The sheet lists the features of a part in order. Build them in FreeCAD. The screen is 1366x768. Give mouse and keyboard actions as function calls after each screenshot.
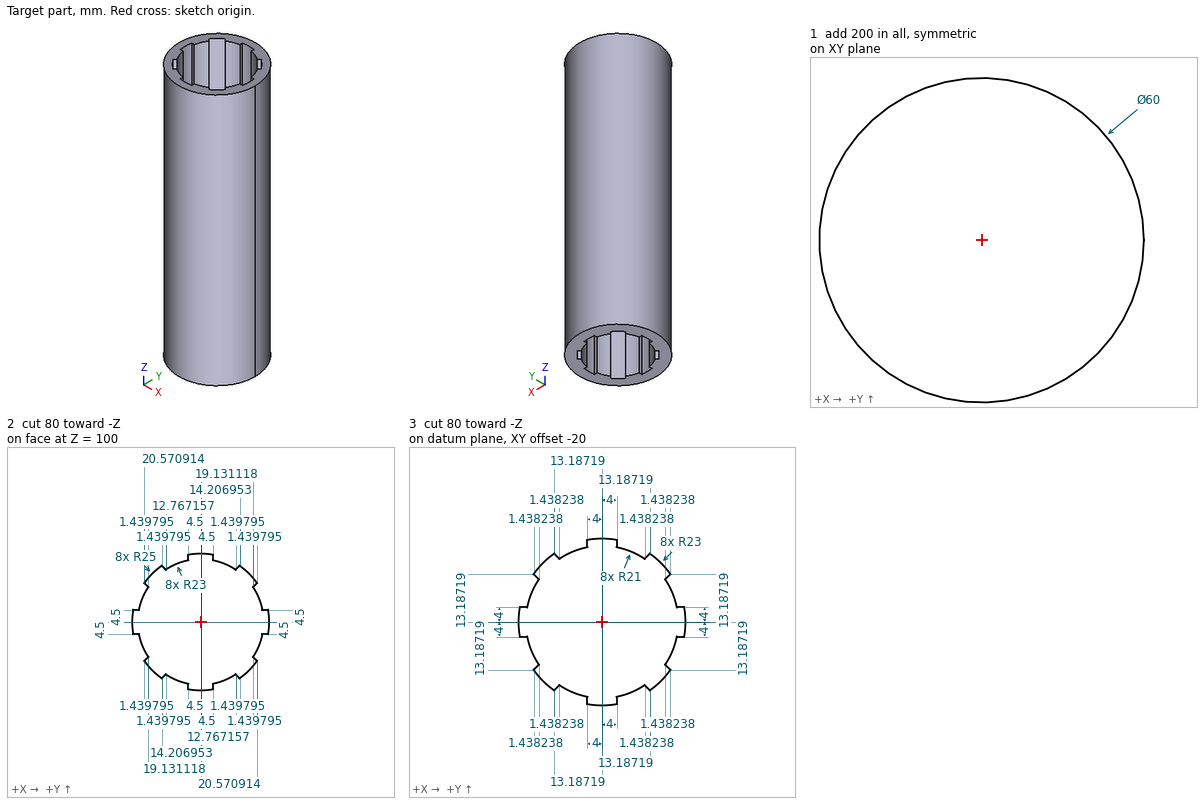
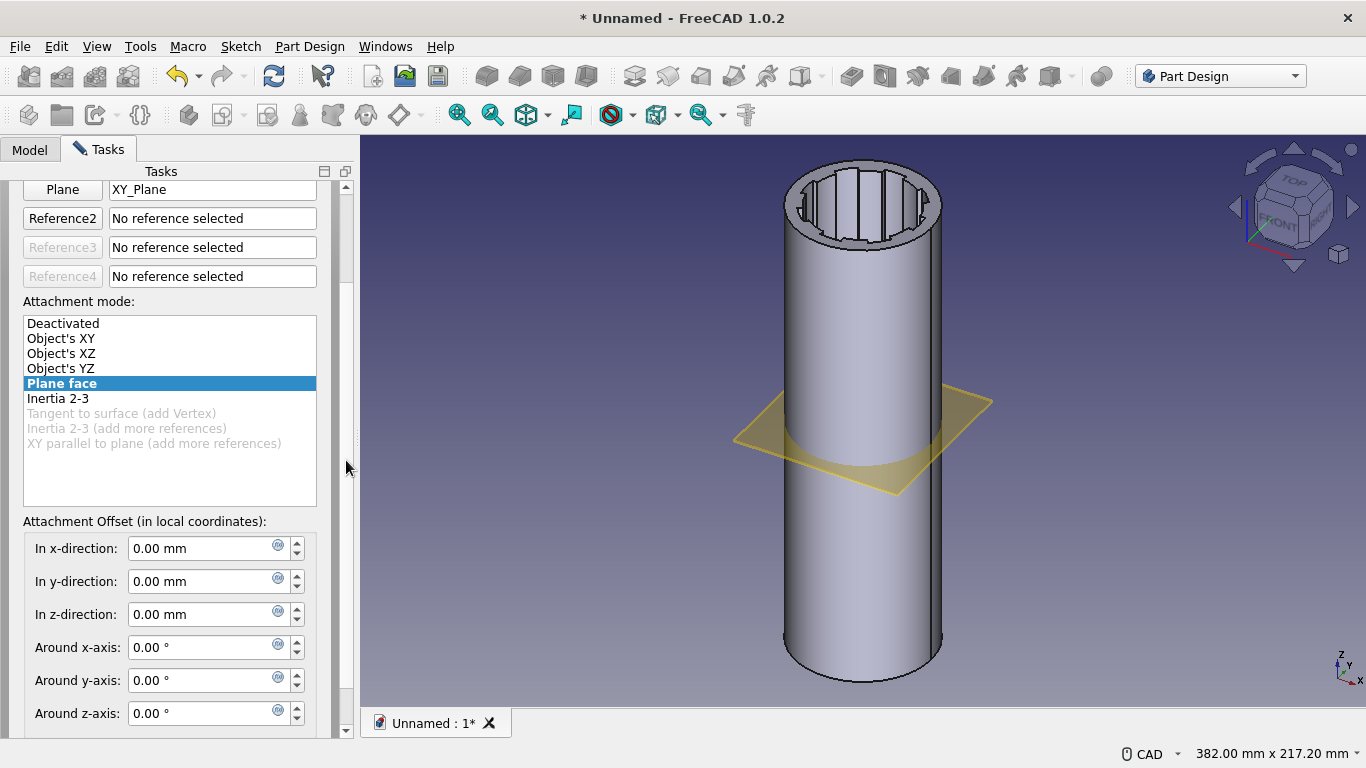
triple_click(210, 614)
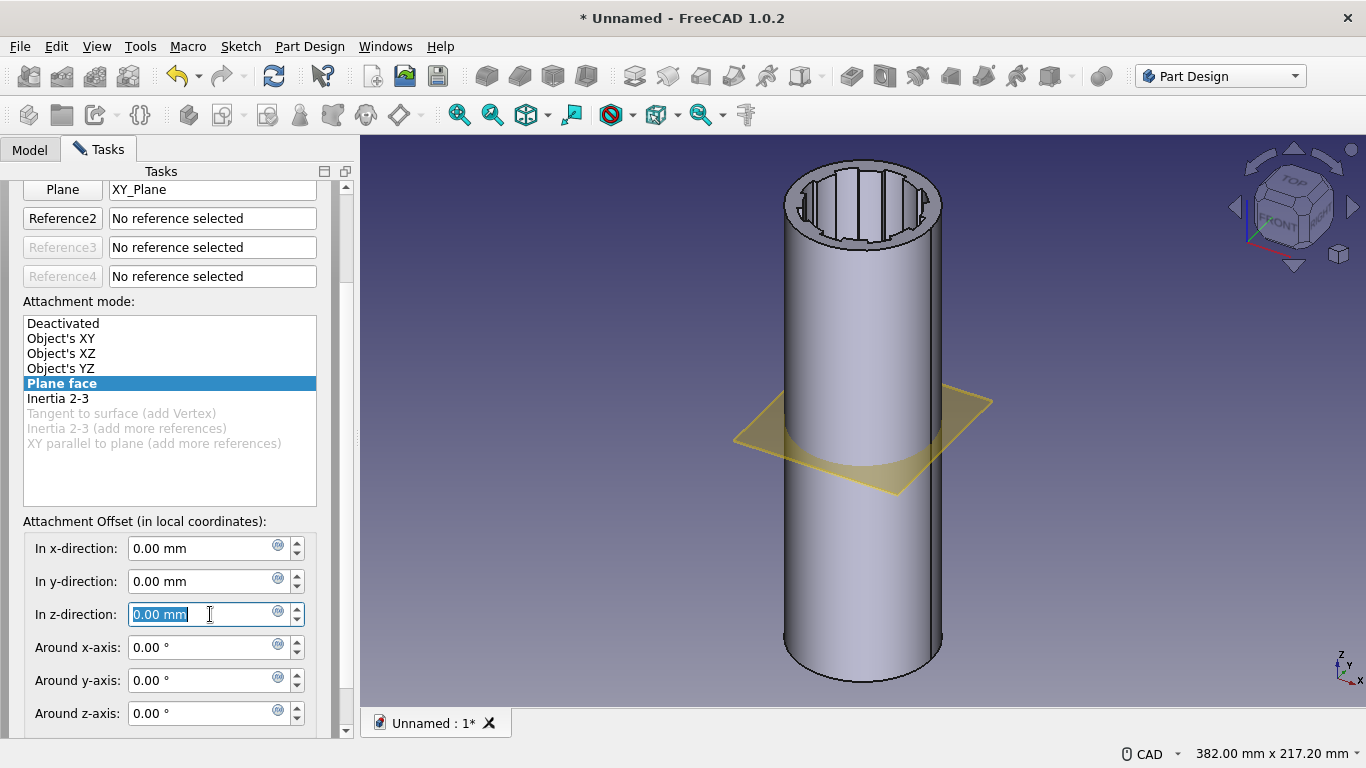
text(-20)
key(Tab)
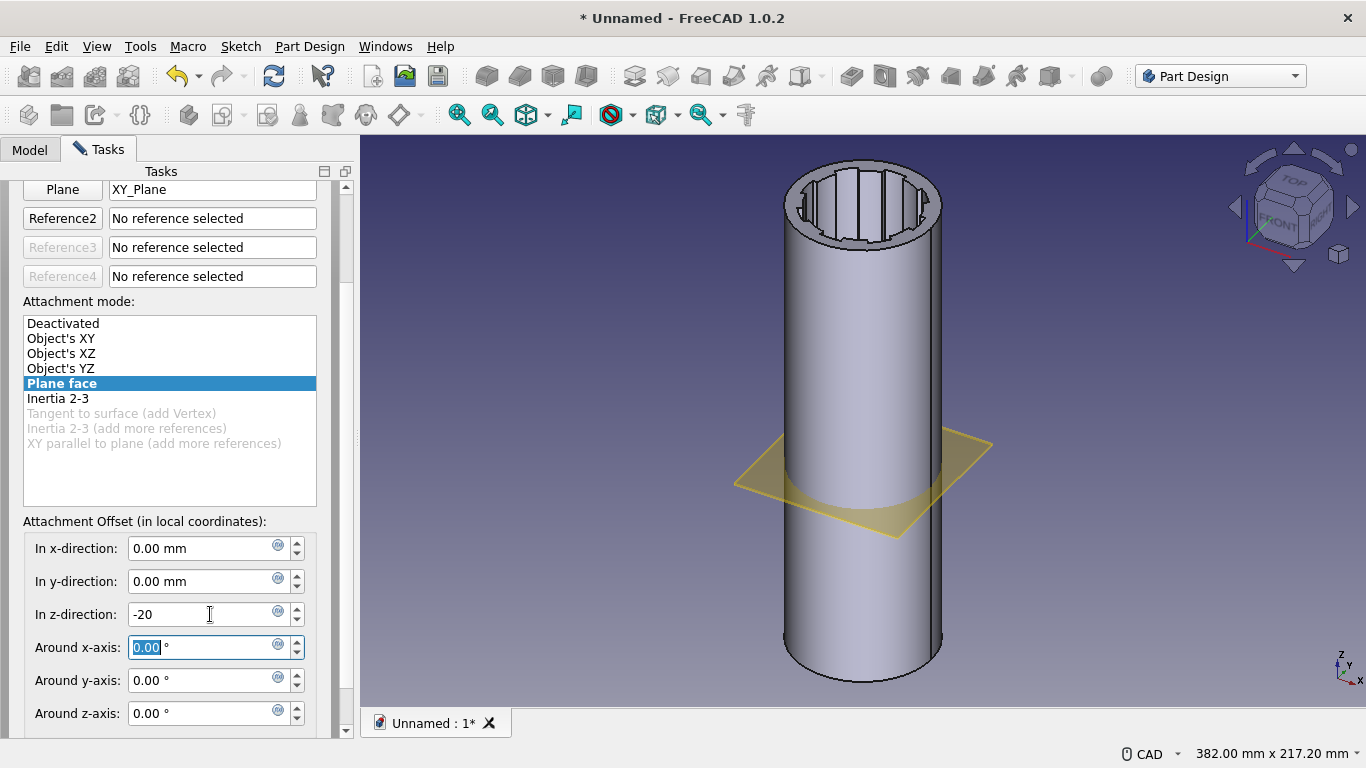
scroll(346, 460, up, 3)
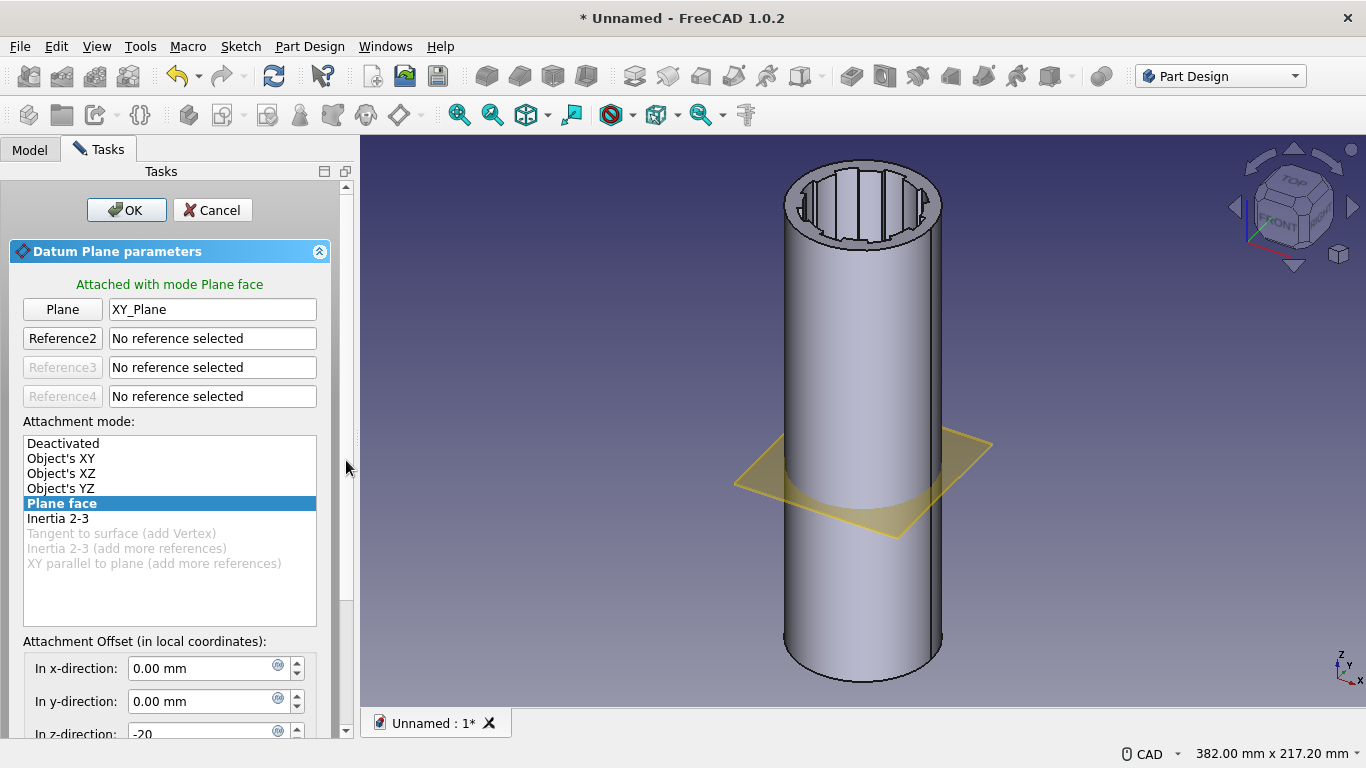
click(127, 210)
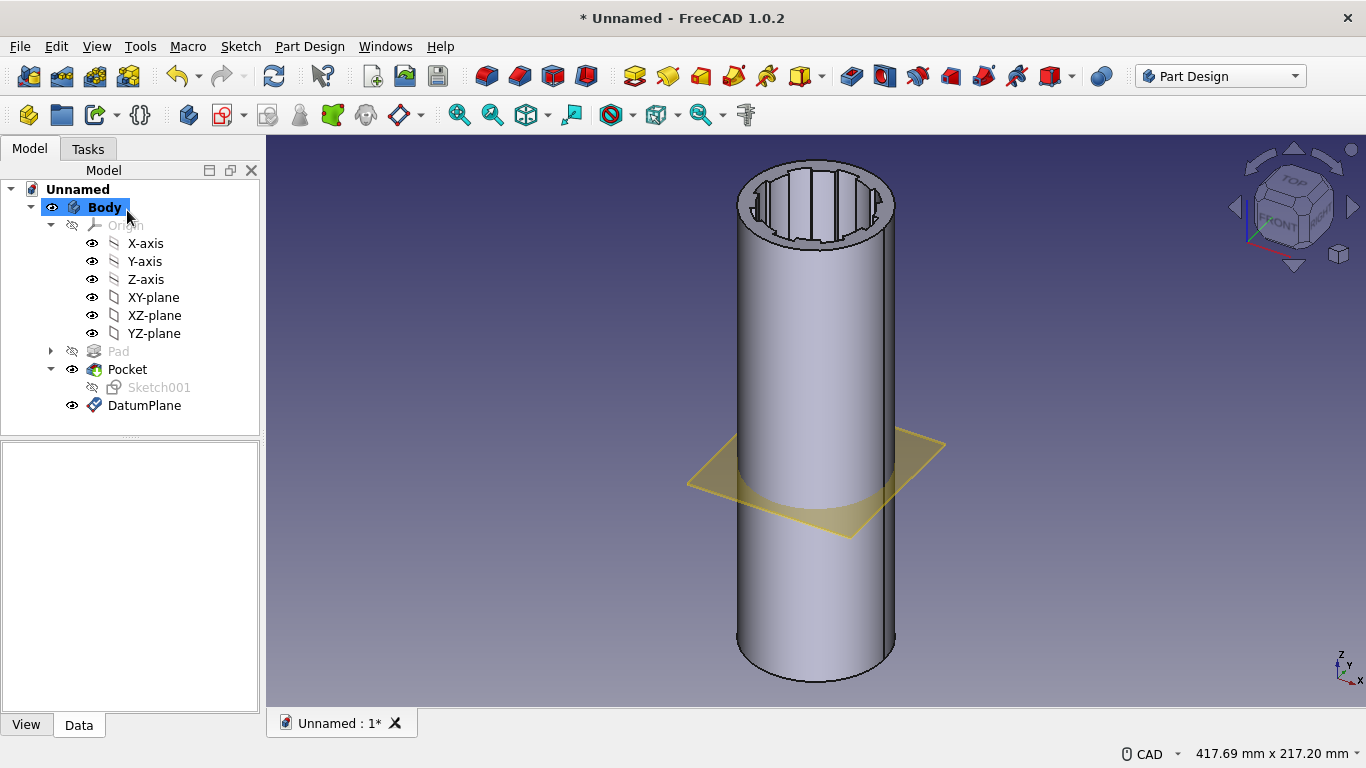
click(117, 405)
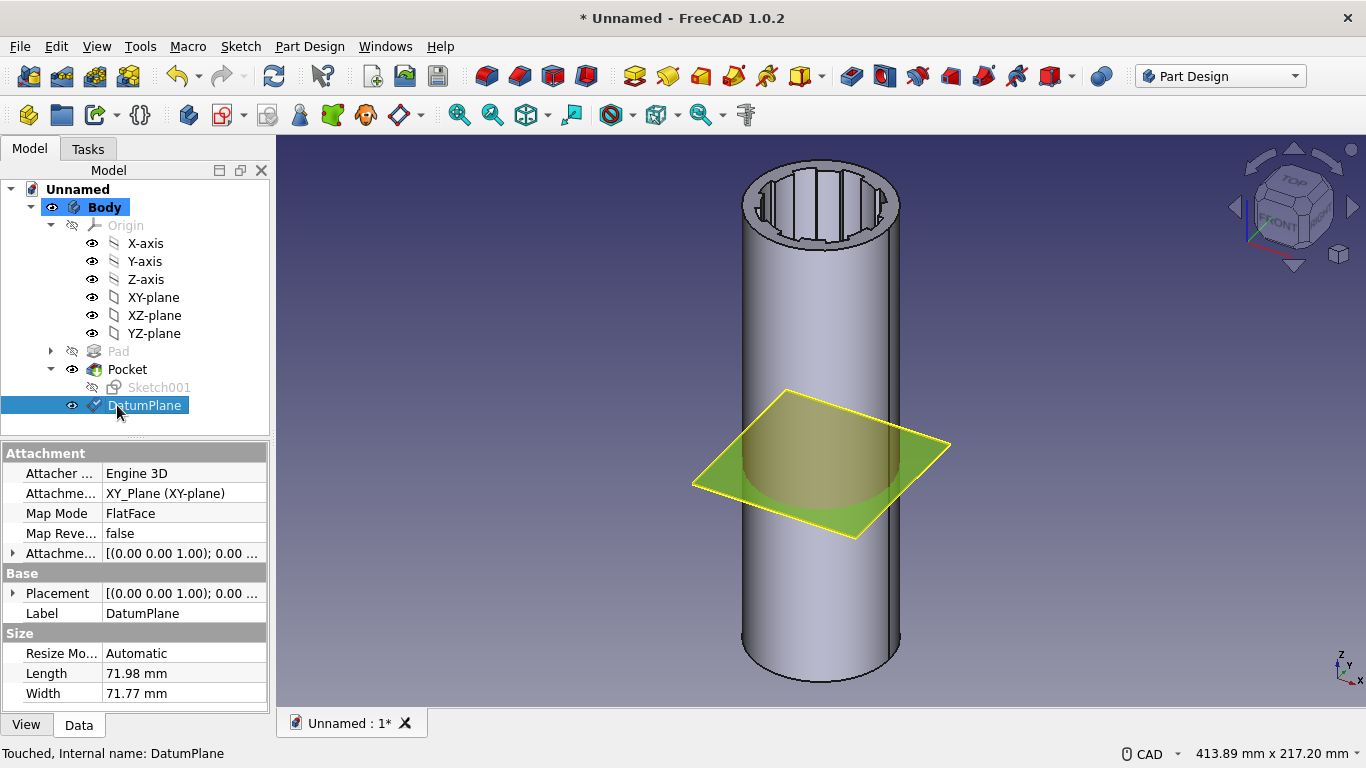
click(222, 116)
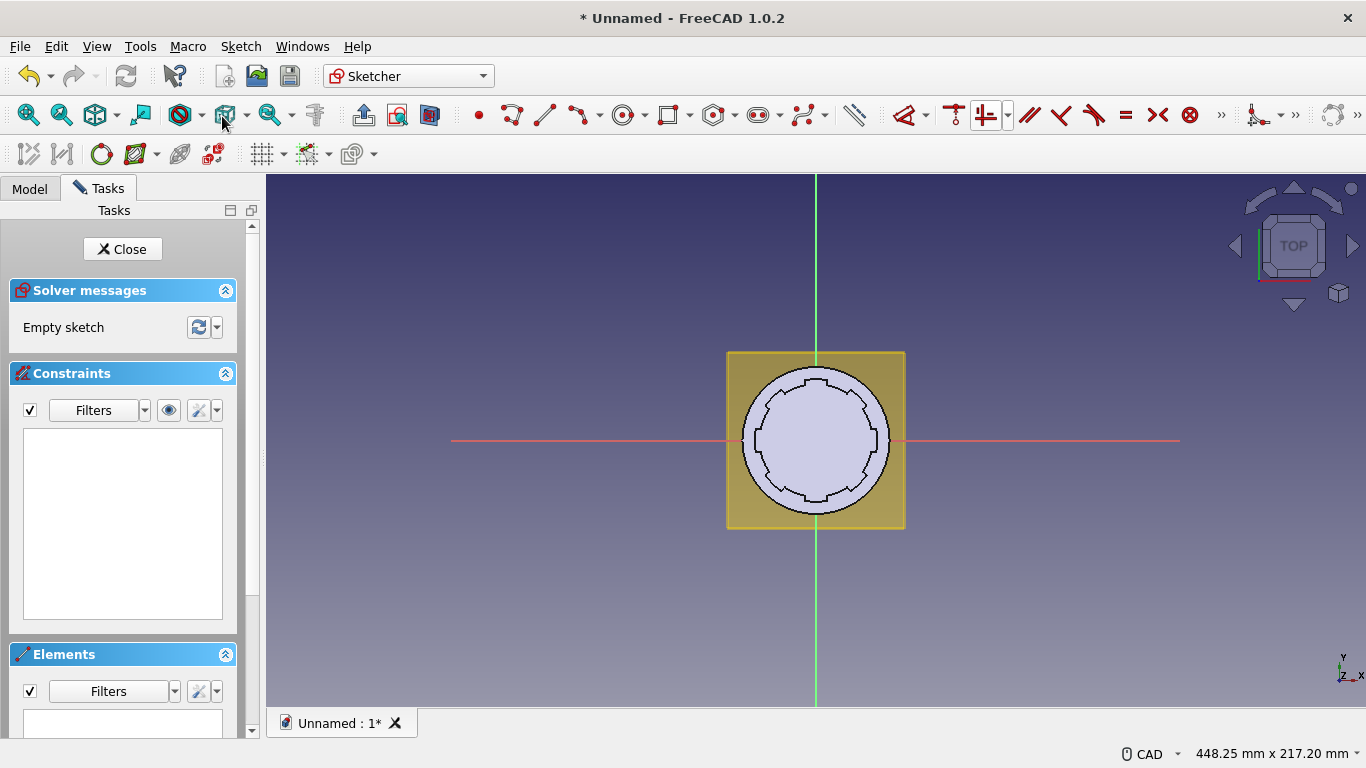
click(430, 116)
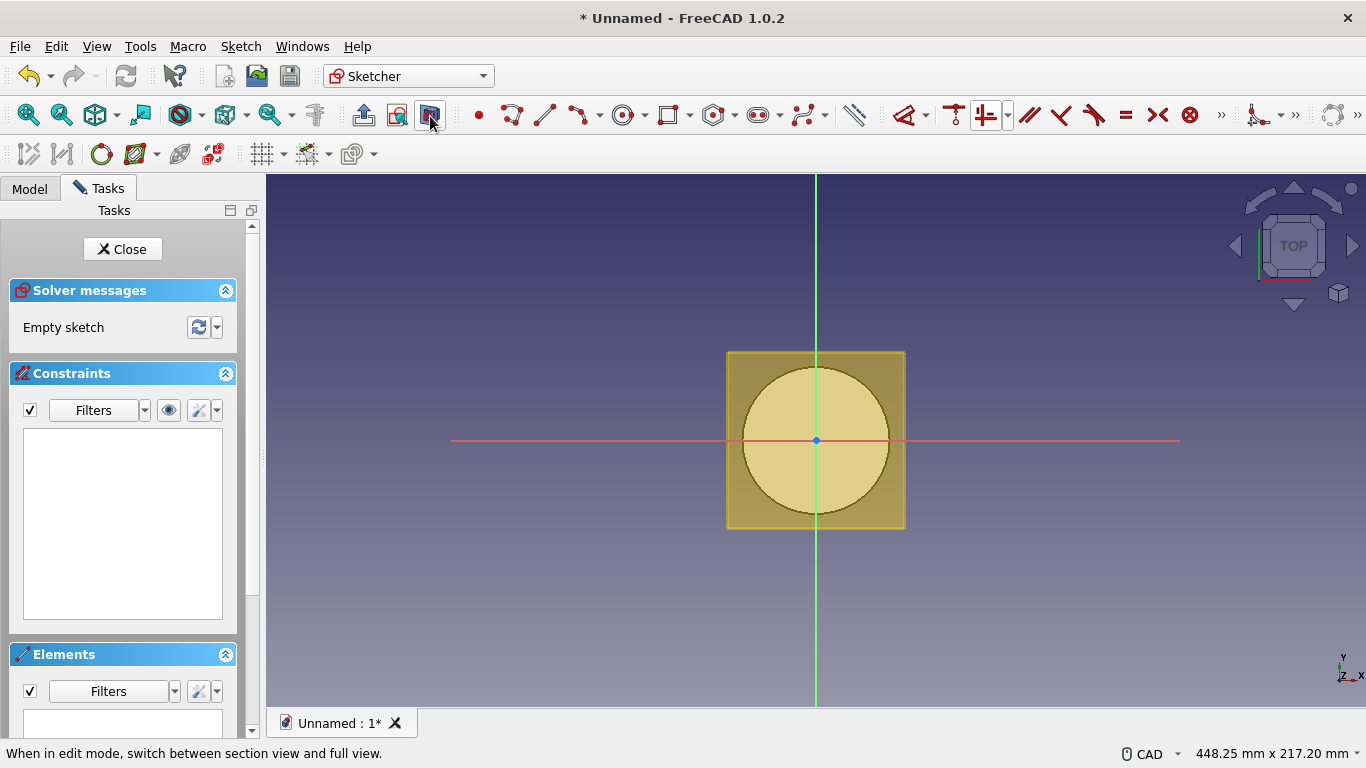
scroll(856, 440, up, 5)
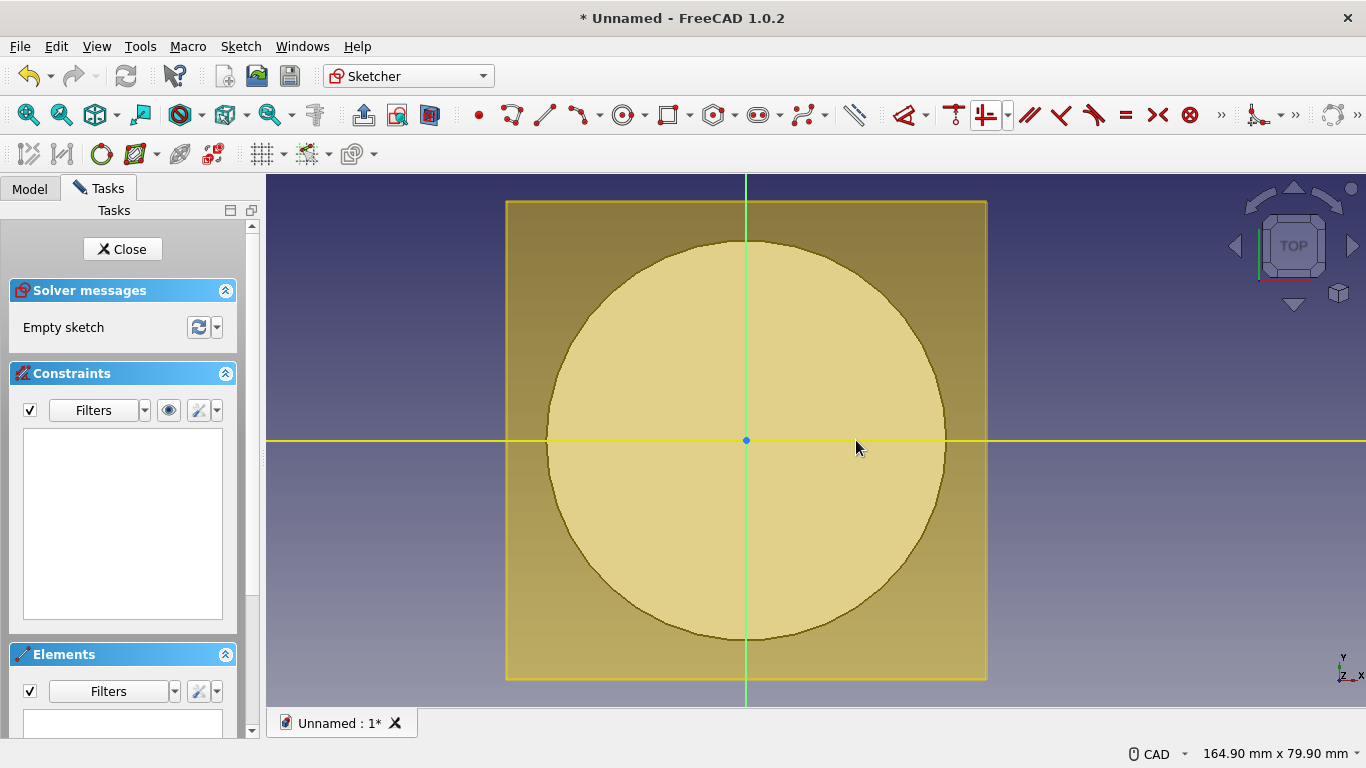
click(545, 116)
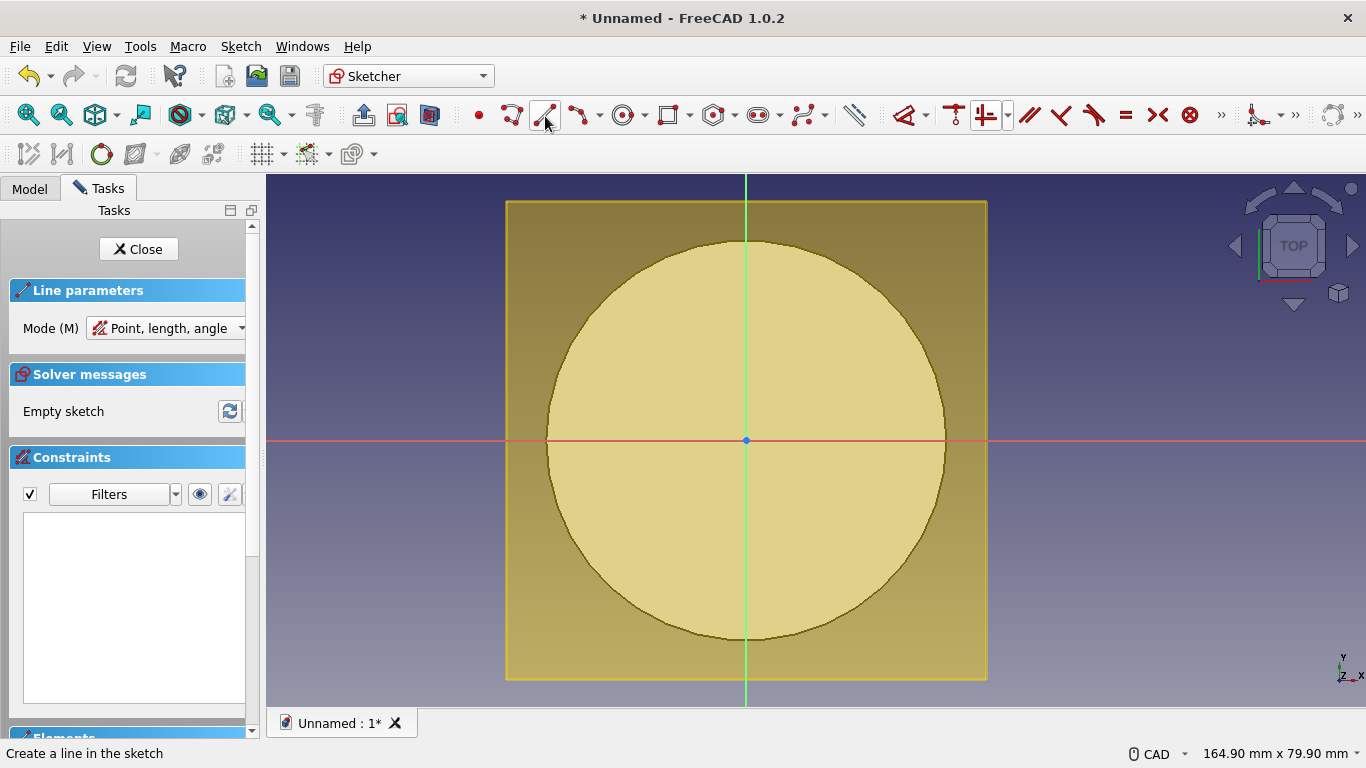
click(773, 289)
click(773, 303)